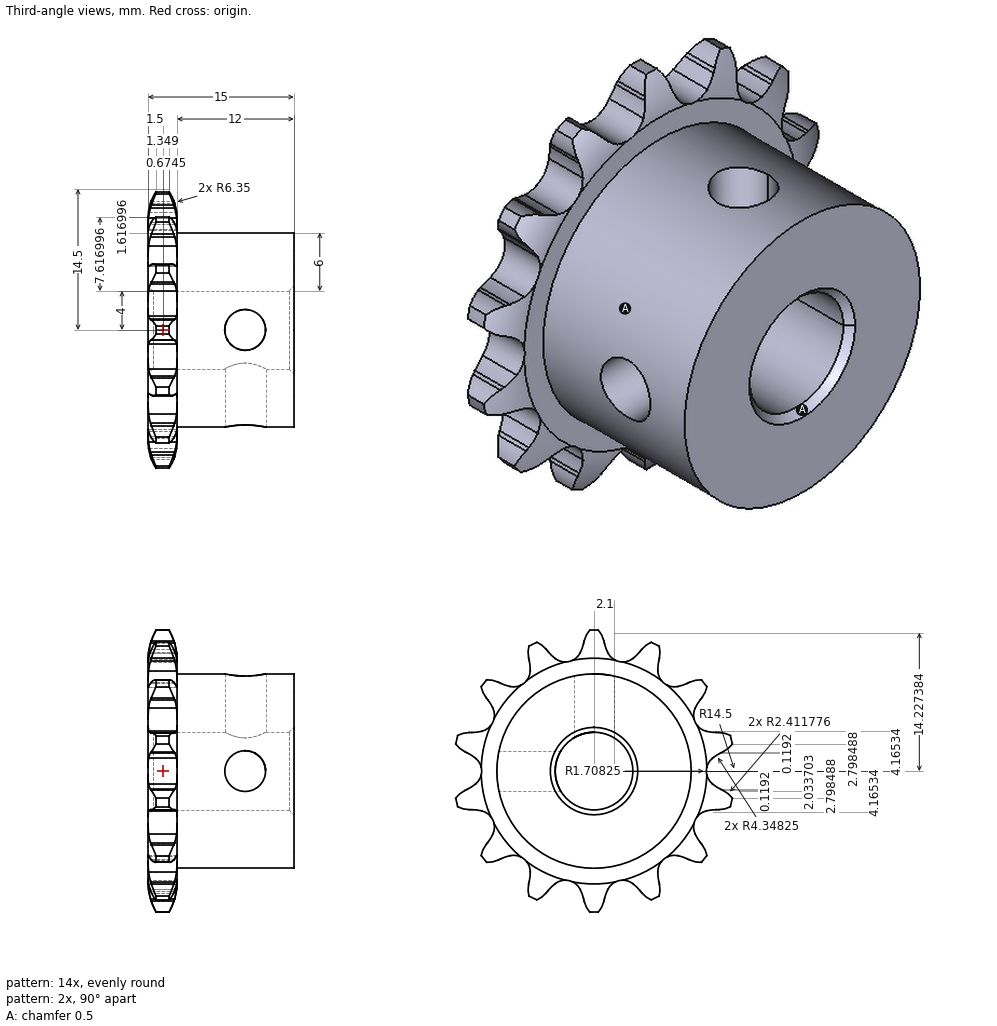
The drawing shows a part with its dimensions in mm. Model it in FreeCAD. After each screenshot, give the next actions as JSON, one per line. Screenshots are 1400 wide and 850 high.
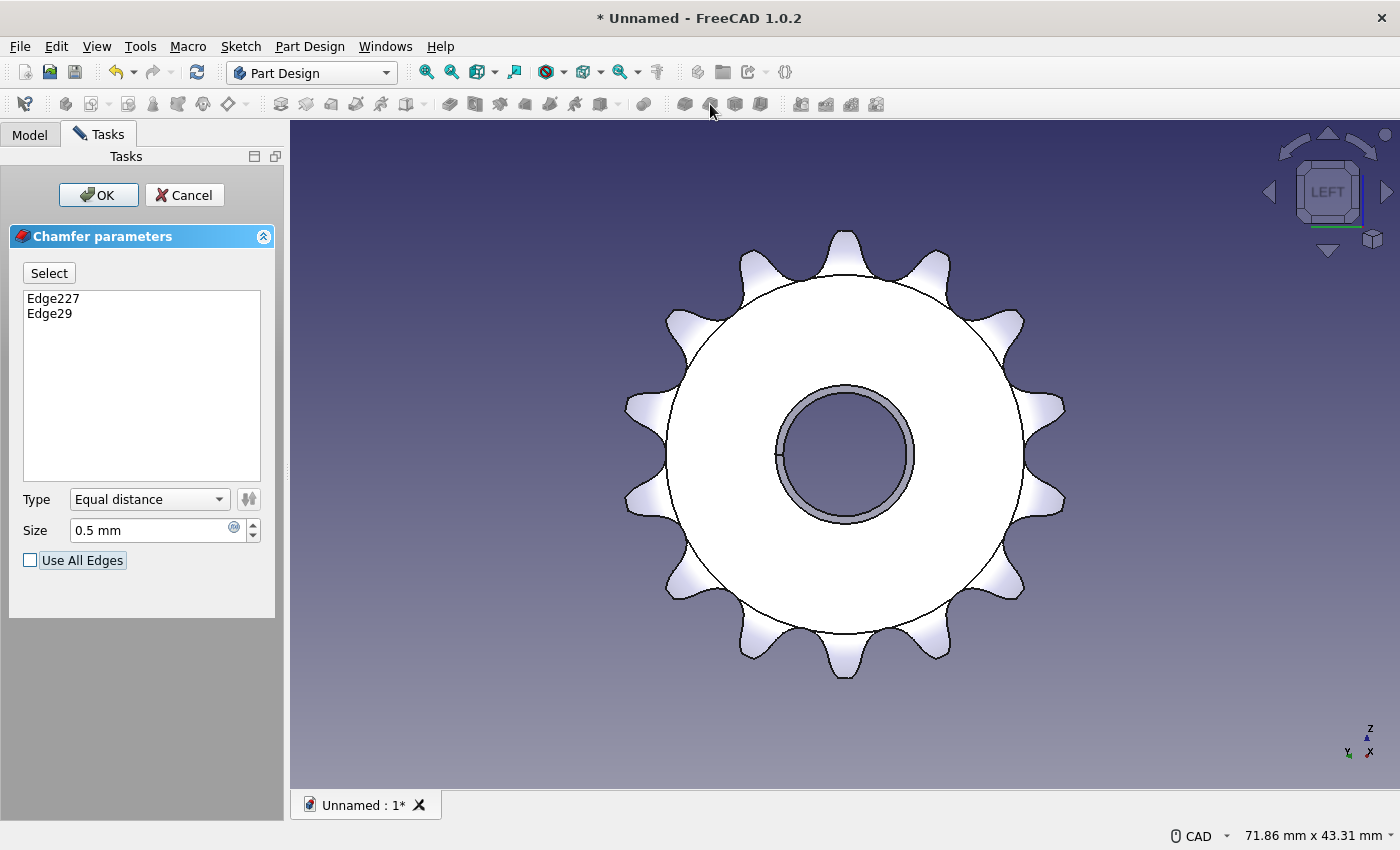
{"action": "left_click", "coordinate": [99, 195]}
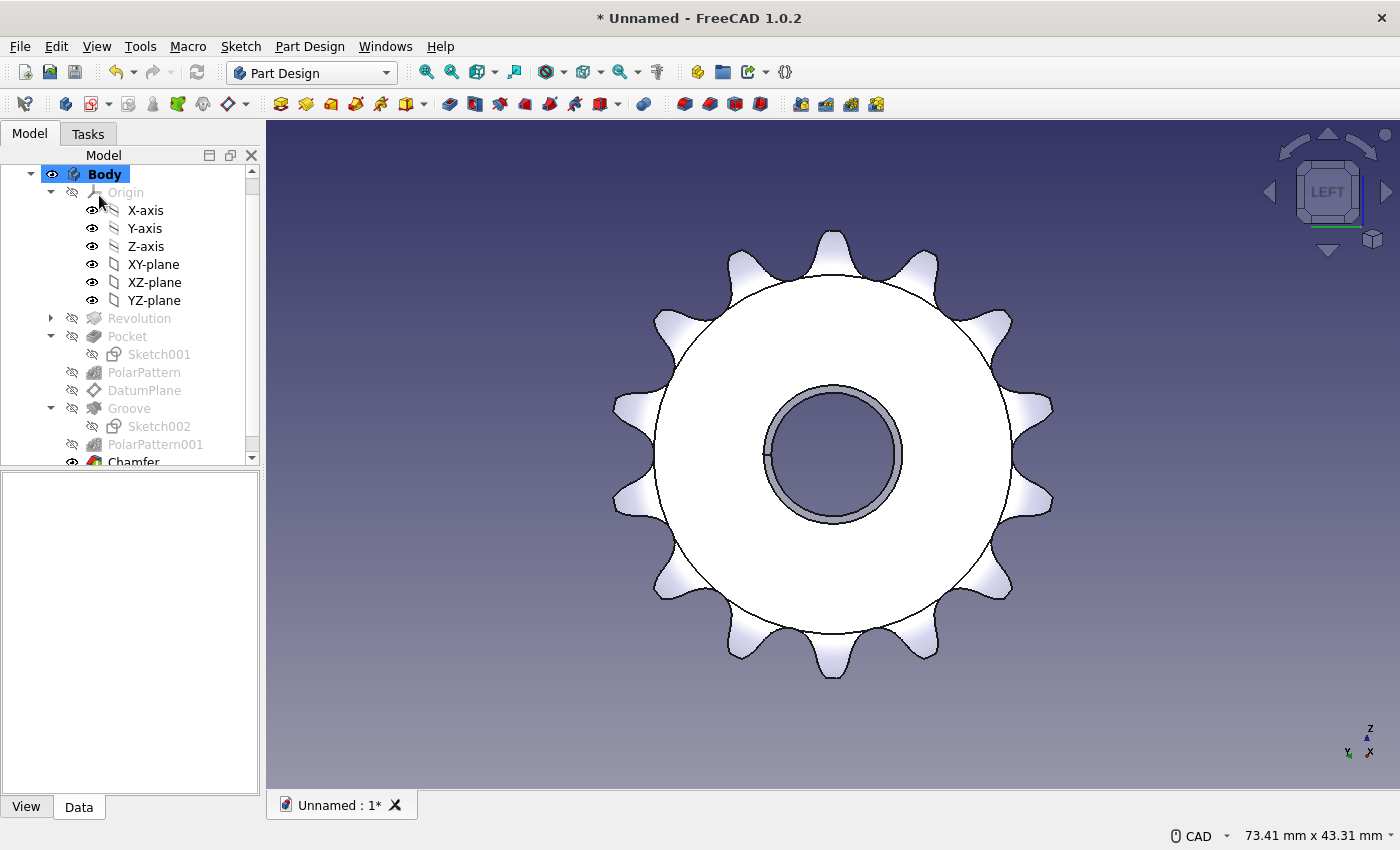
{"action": "key", "text": "0"}